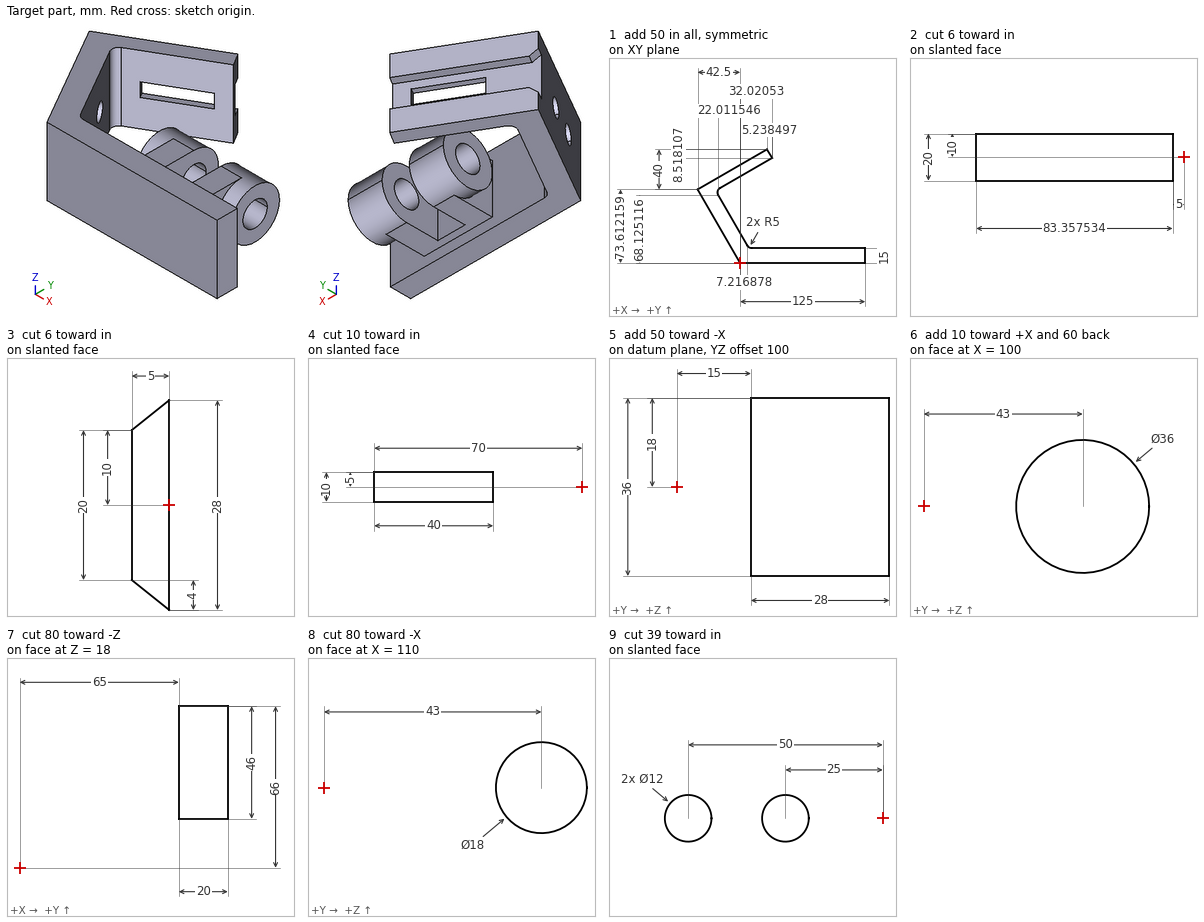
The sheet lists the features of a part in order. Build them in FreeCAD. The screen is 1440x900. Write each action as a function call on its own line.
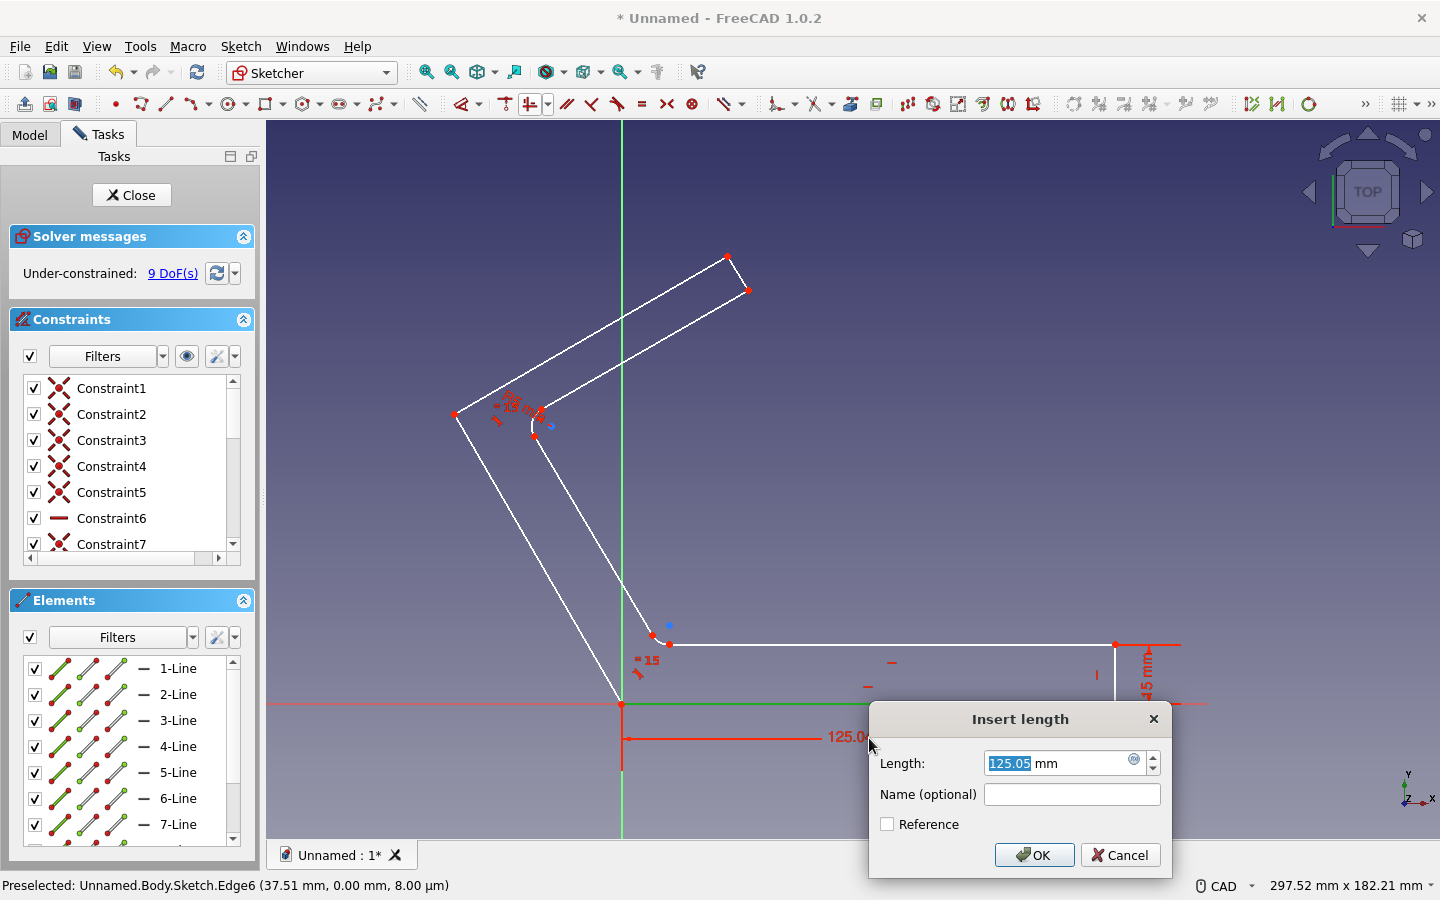
text(125)
key(Return)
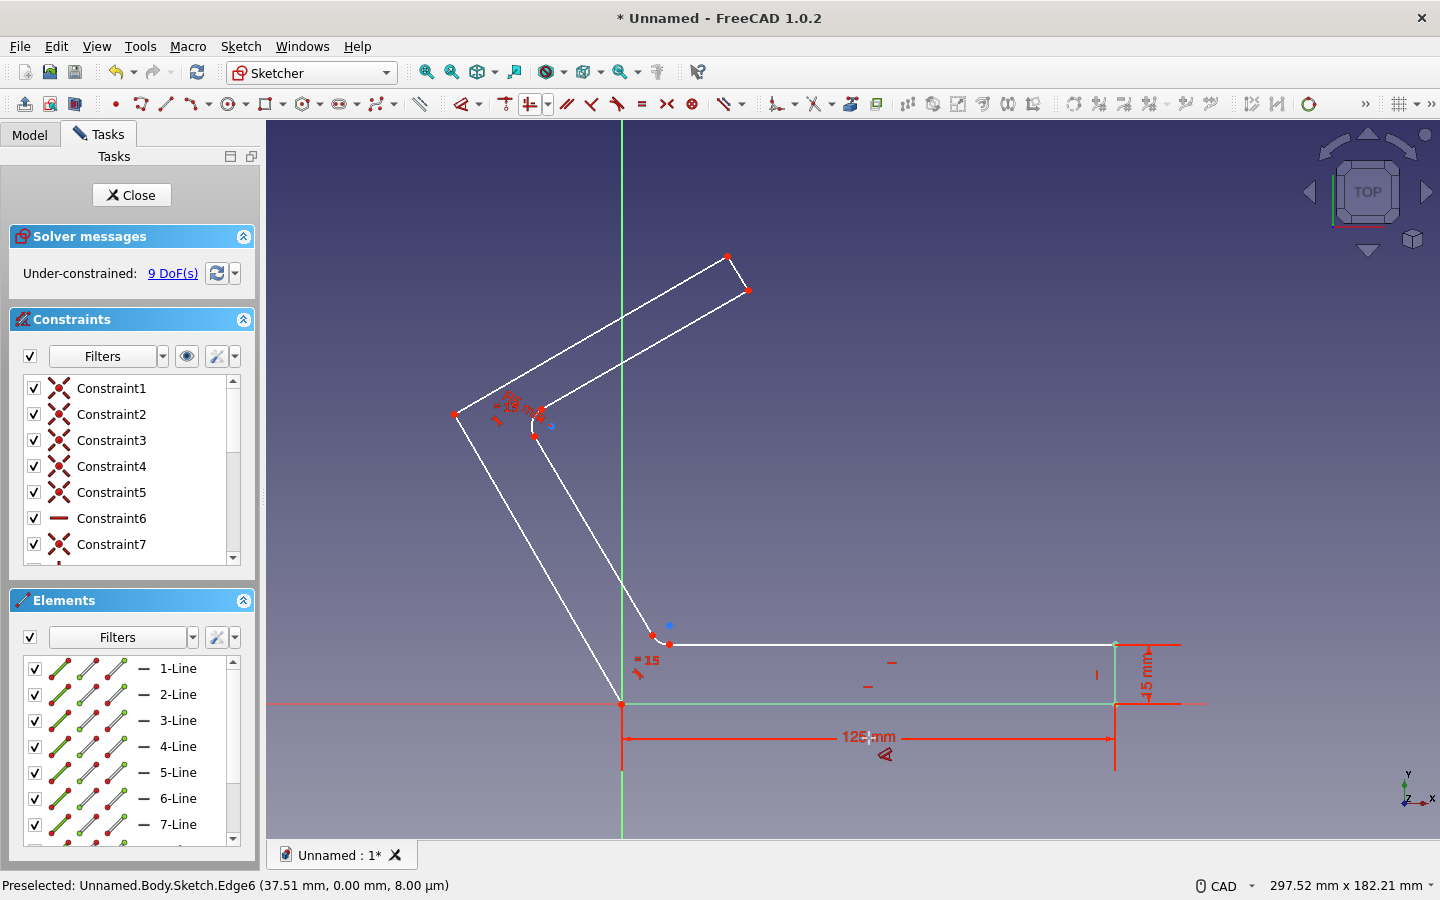
click(646, 304)
click(420, 336)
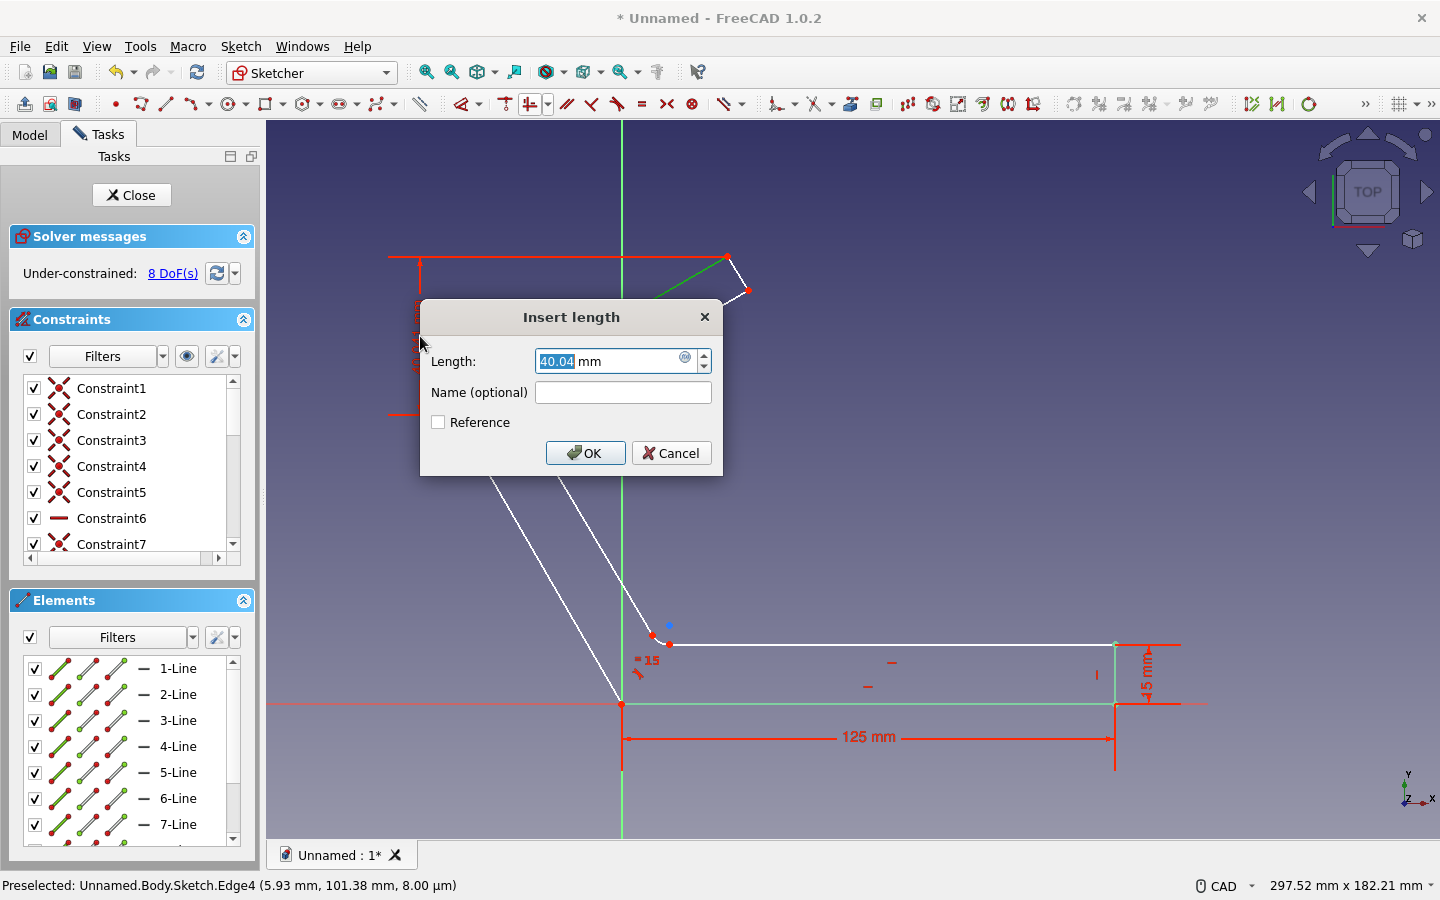
text(40)
key(Return)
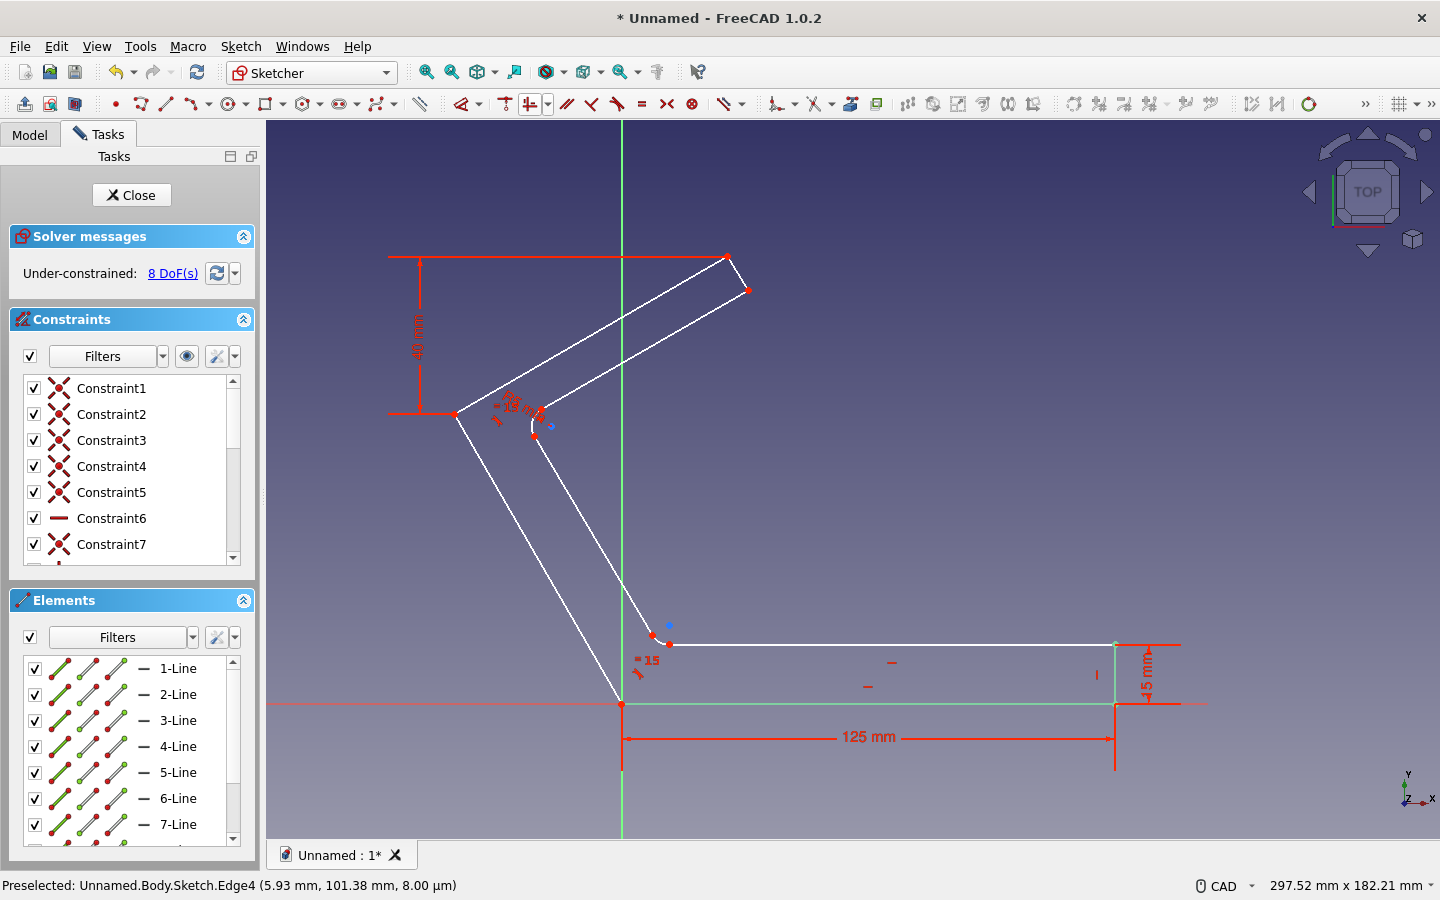
click(454, 414)
click(538, 738)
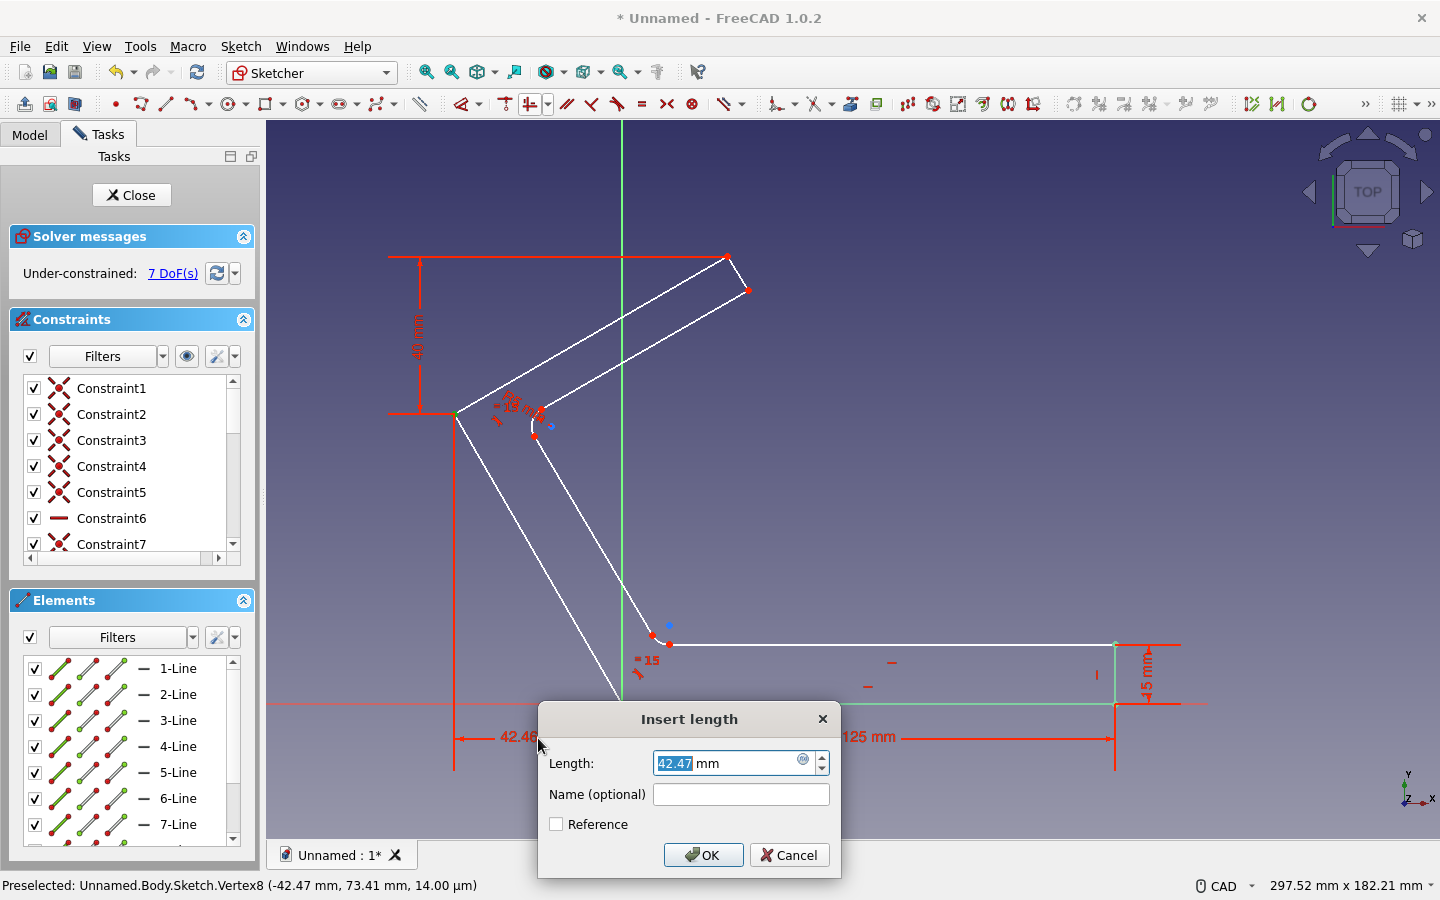
text(42.5)
key(Return)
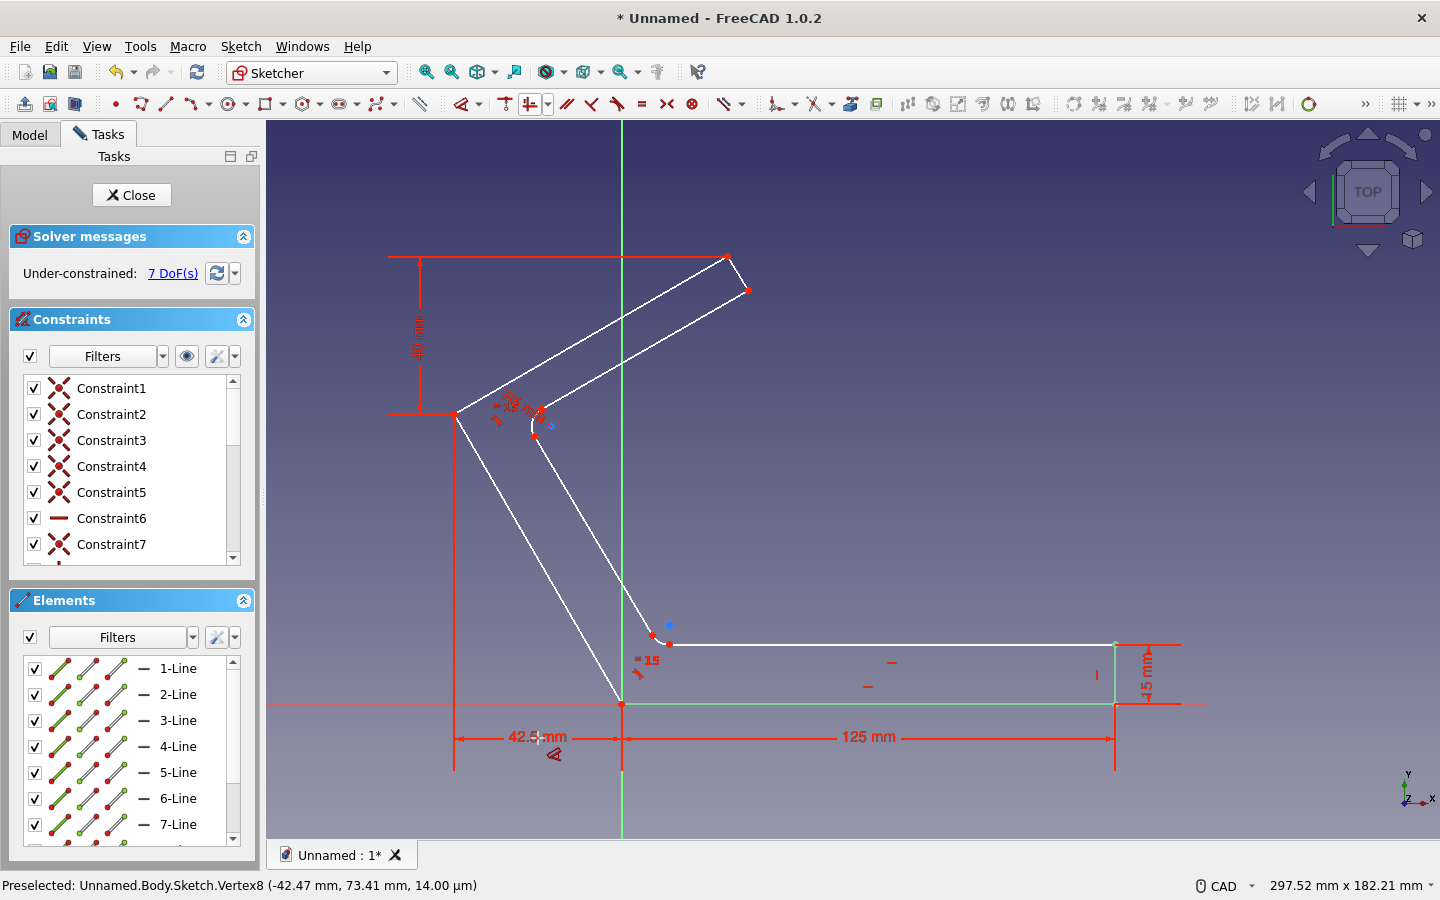
scroll(652, 635, up, 2)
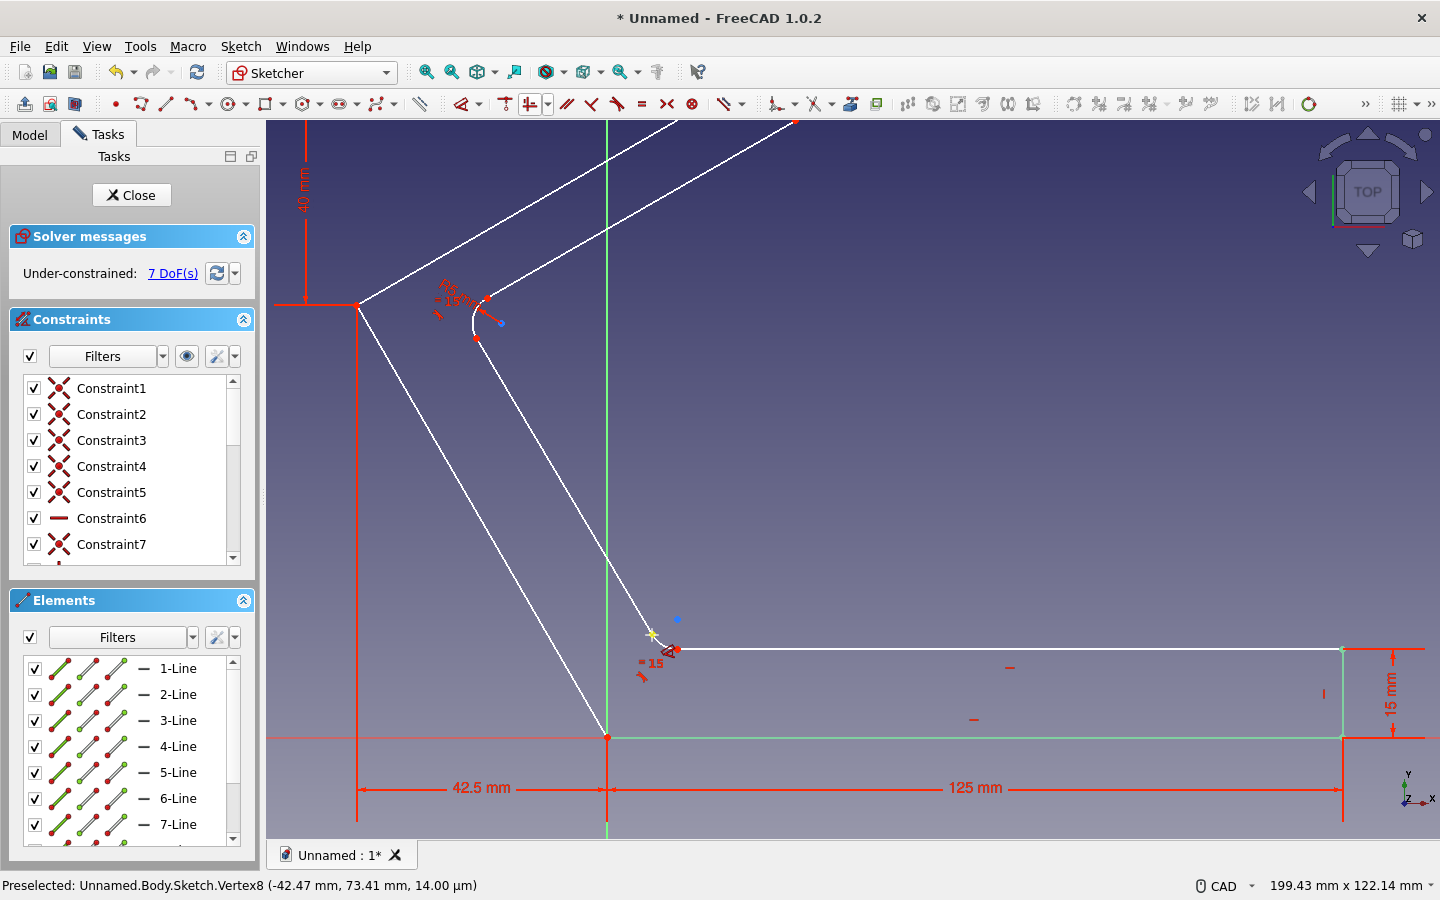
click(652, 635)
click(630, 772)